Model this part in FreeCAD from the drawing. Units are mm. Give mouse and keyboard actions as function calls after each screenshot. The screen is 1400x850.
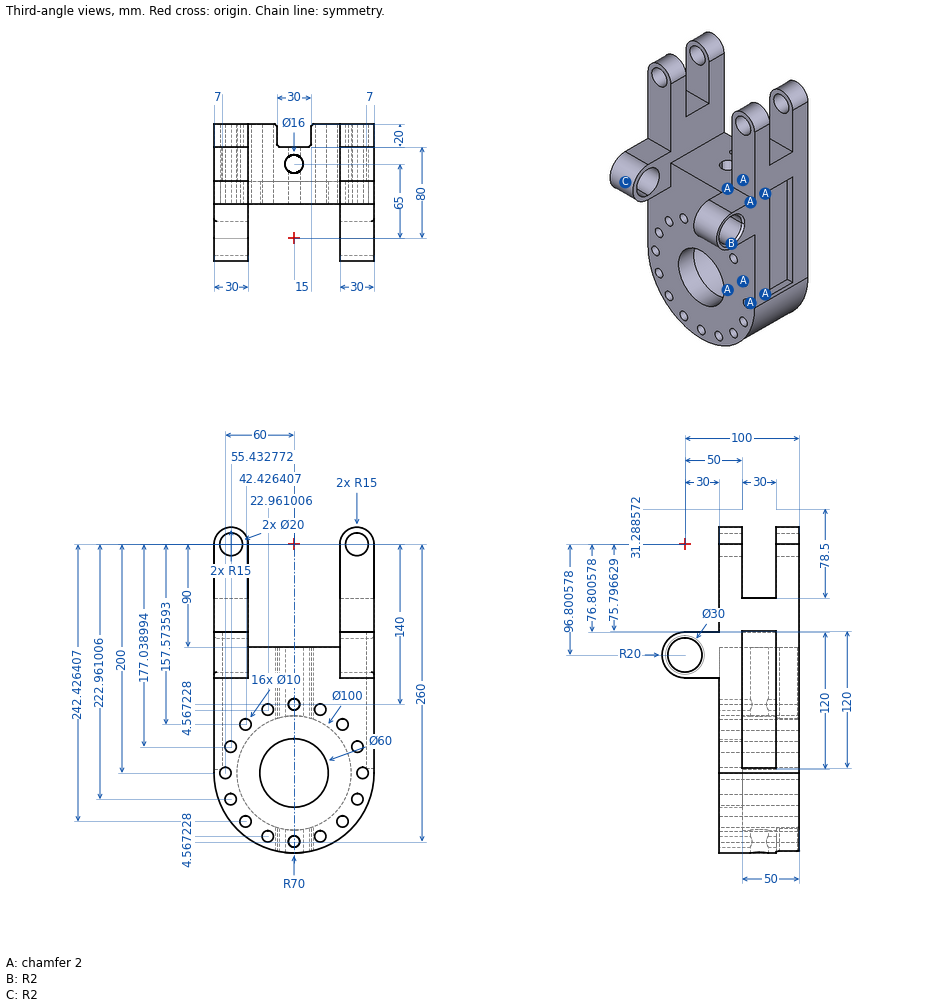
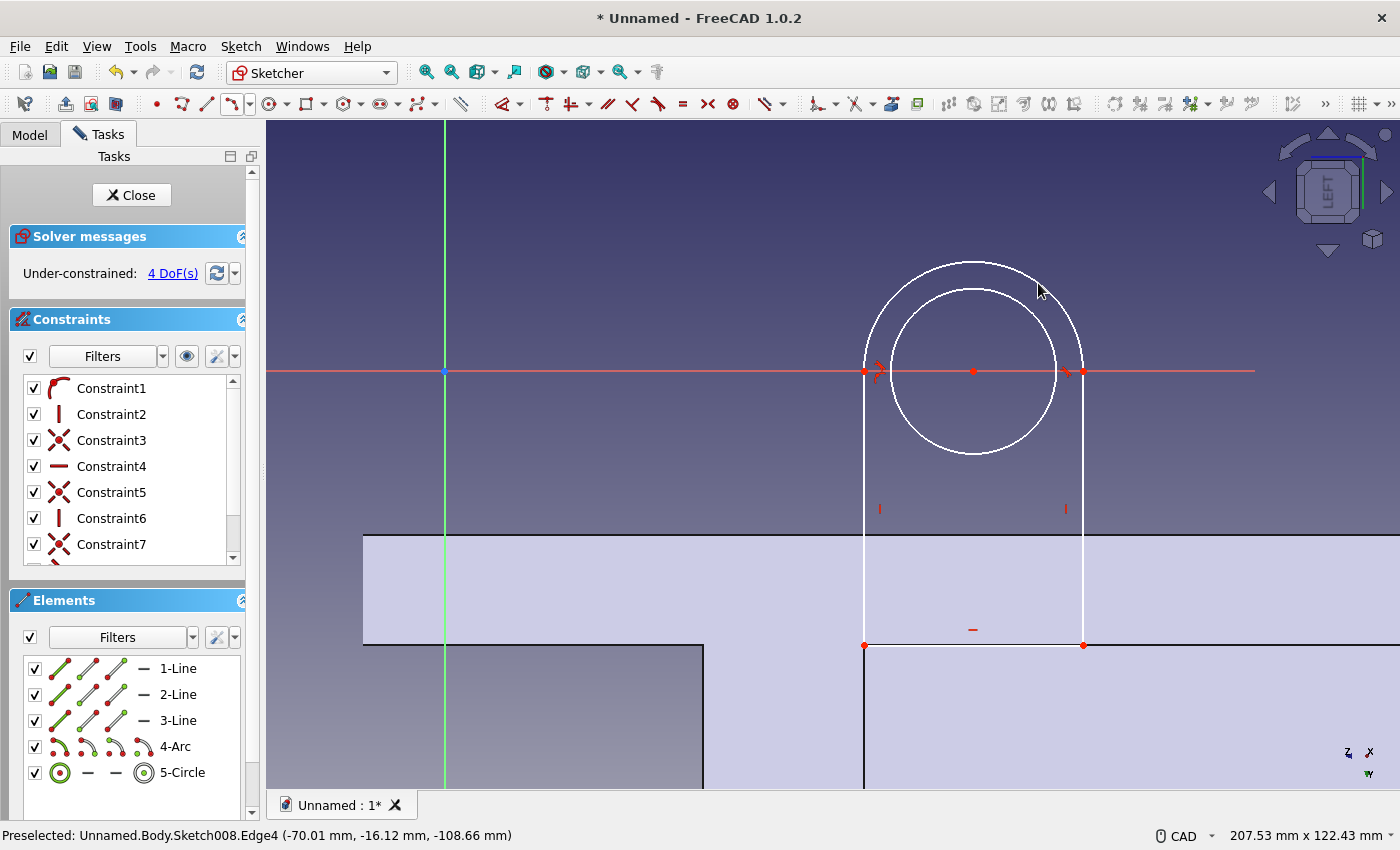
click(502, 104)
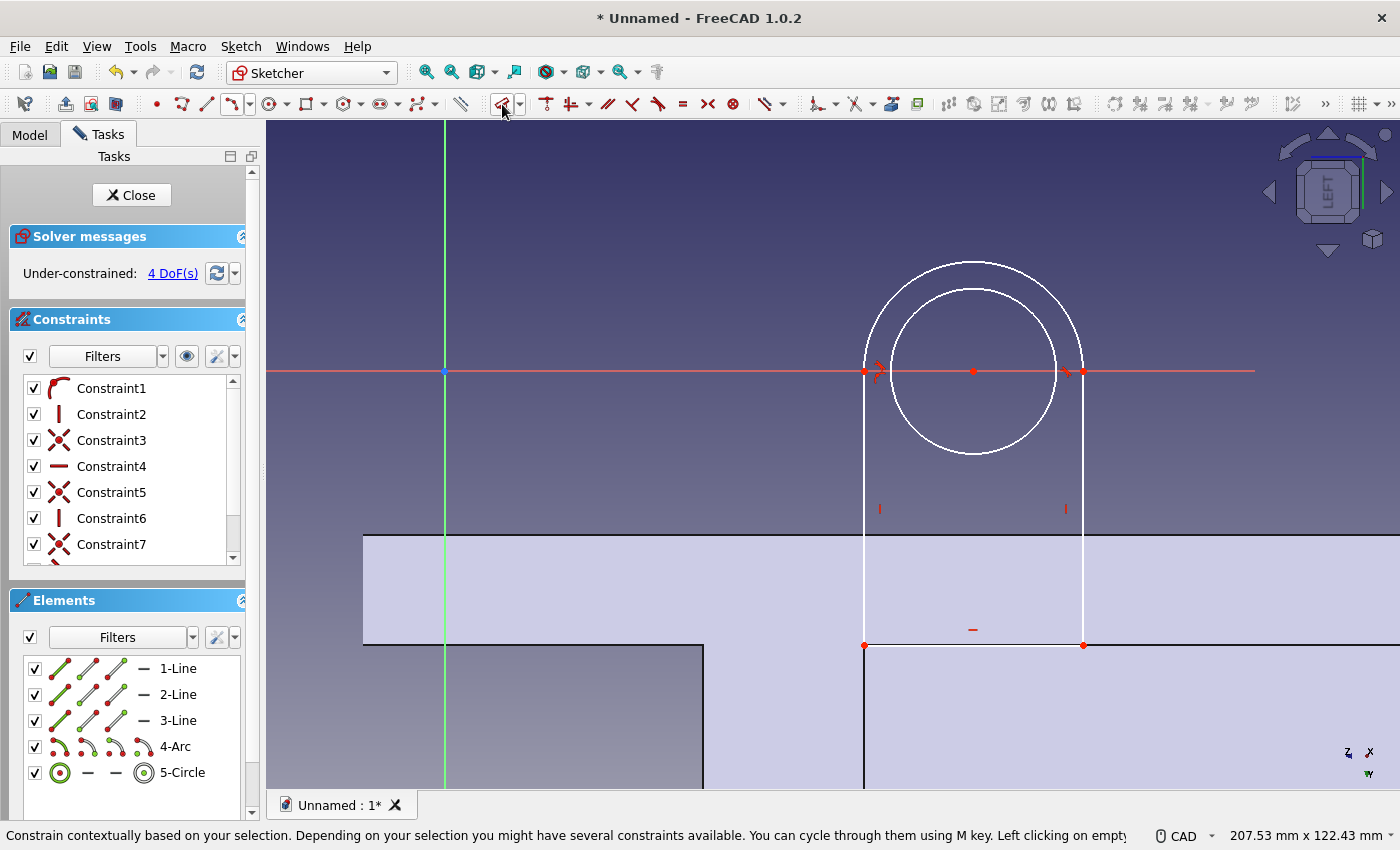
click(1038, 283)
click(1057, 257)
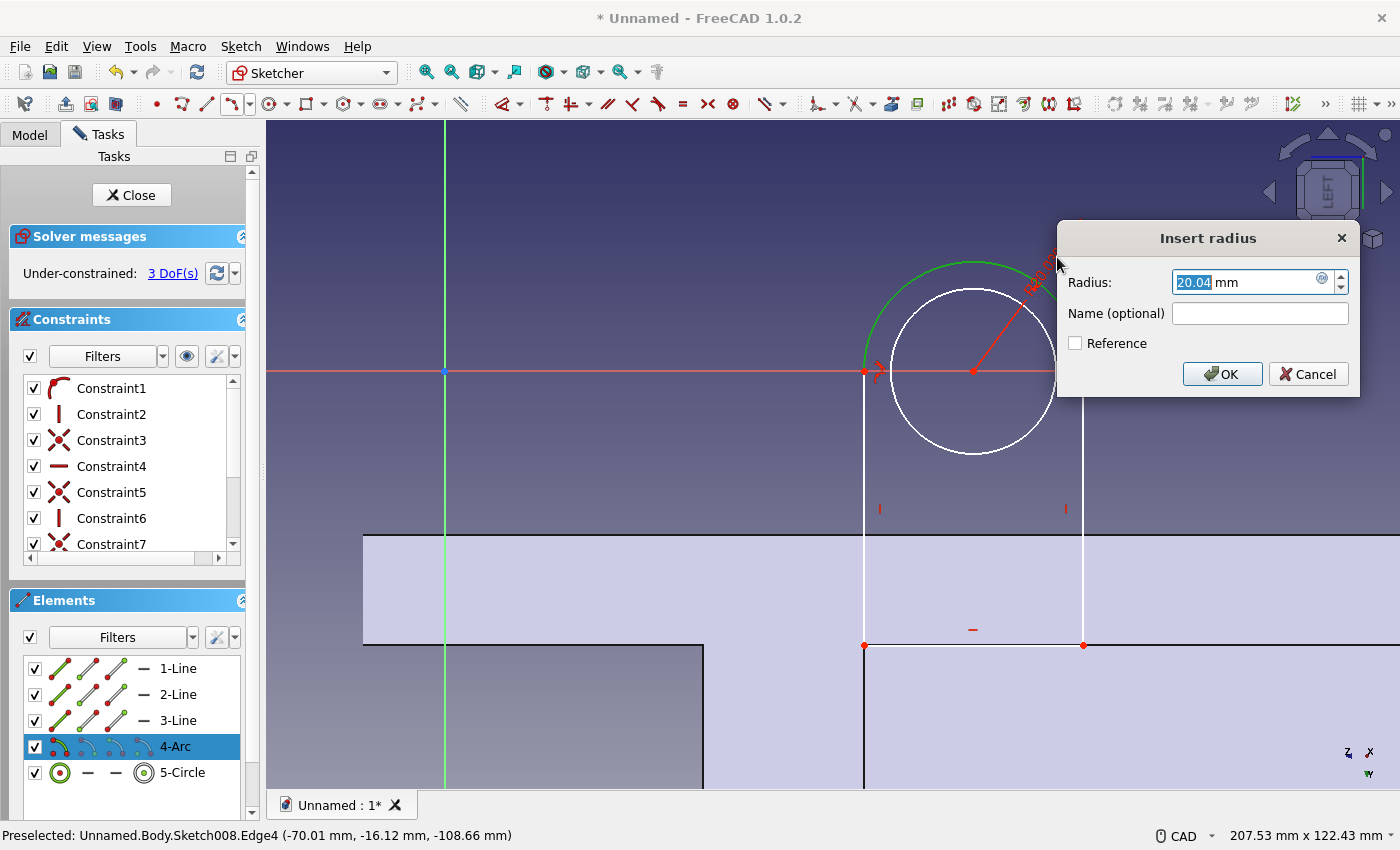
text(20)
key(Return)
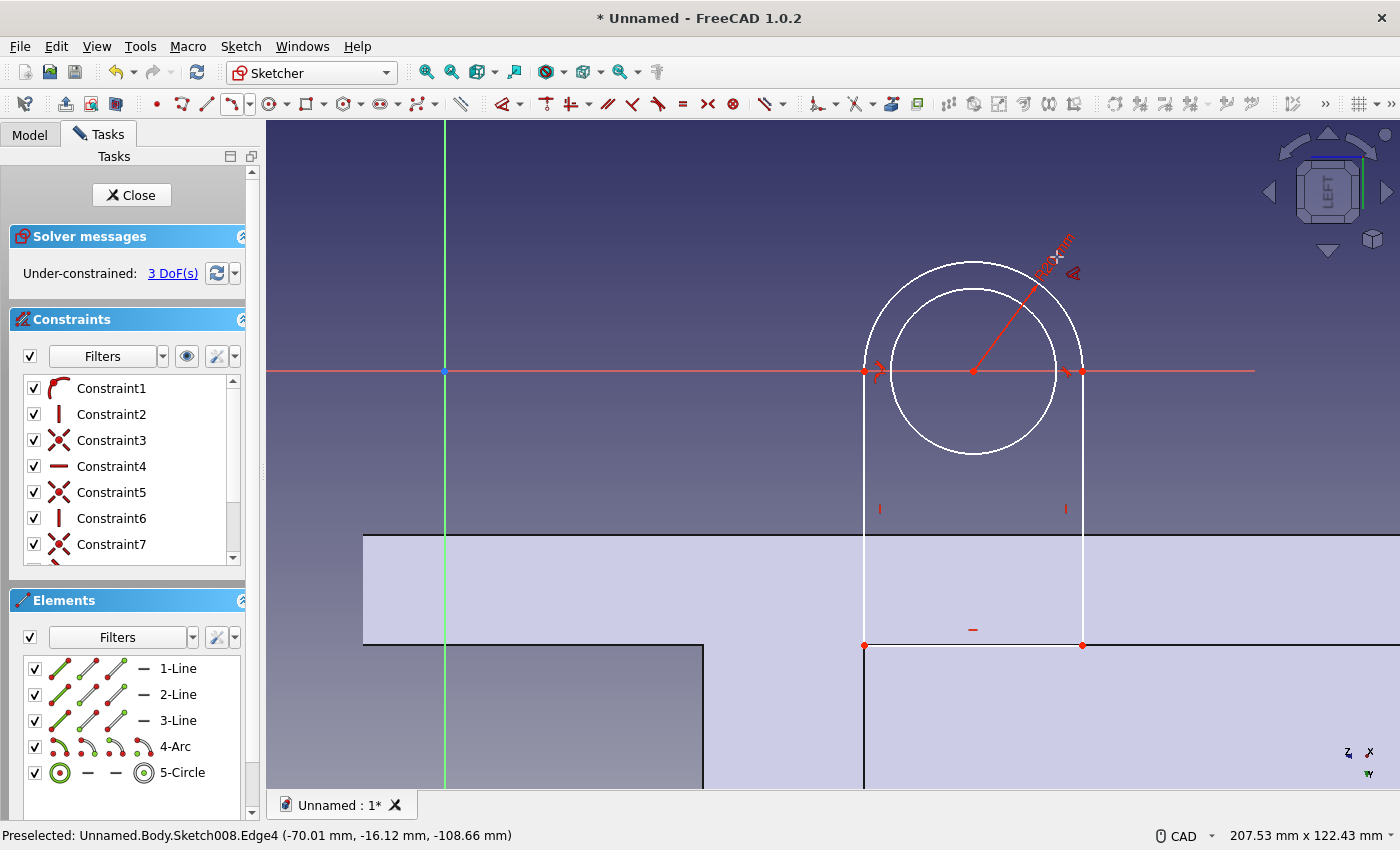
click(1032, 313)
click(1055, 452)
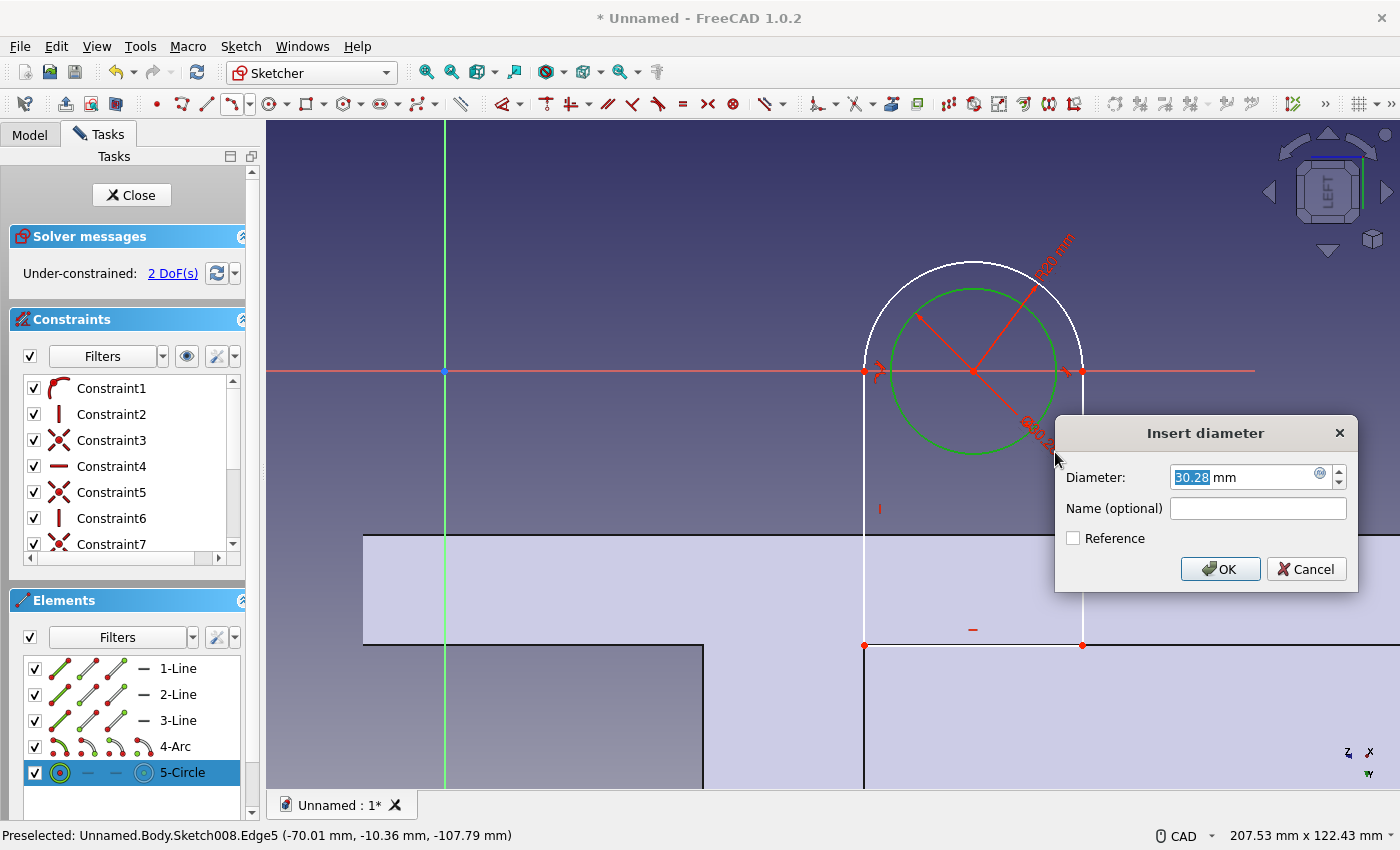
text(30)
key(Return)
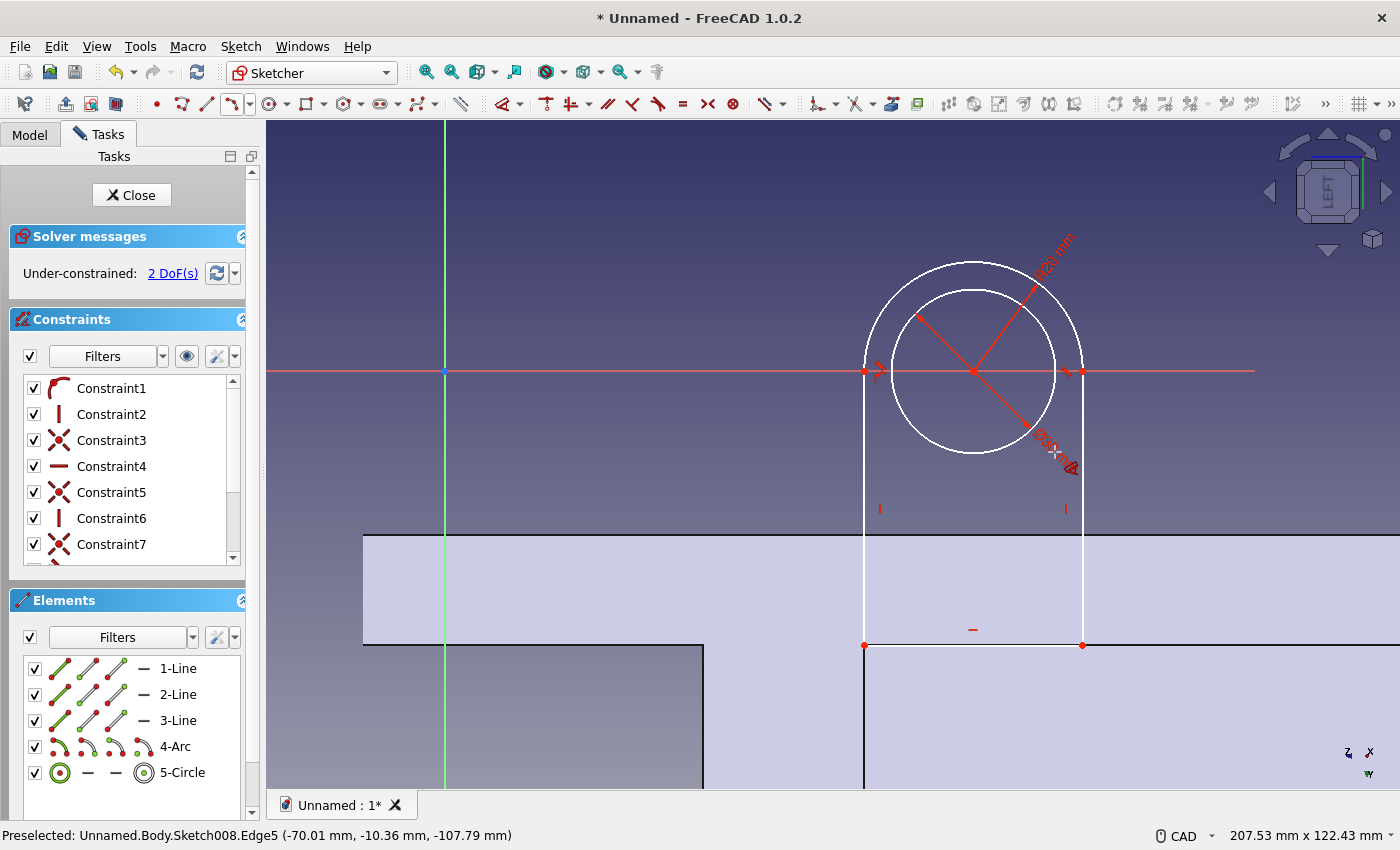
click(864, 454)
click(898, 509)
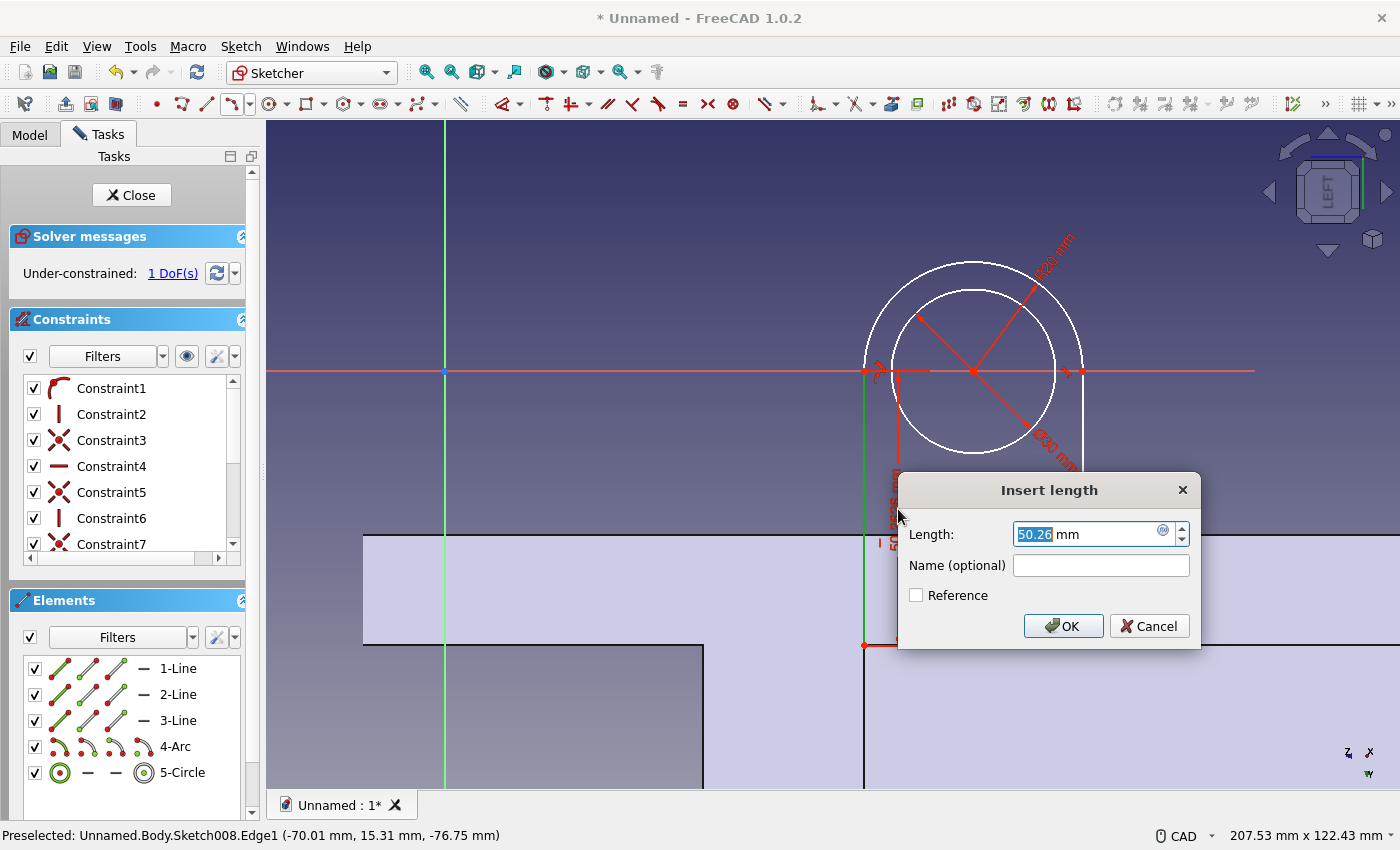
text(50)
key(Return)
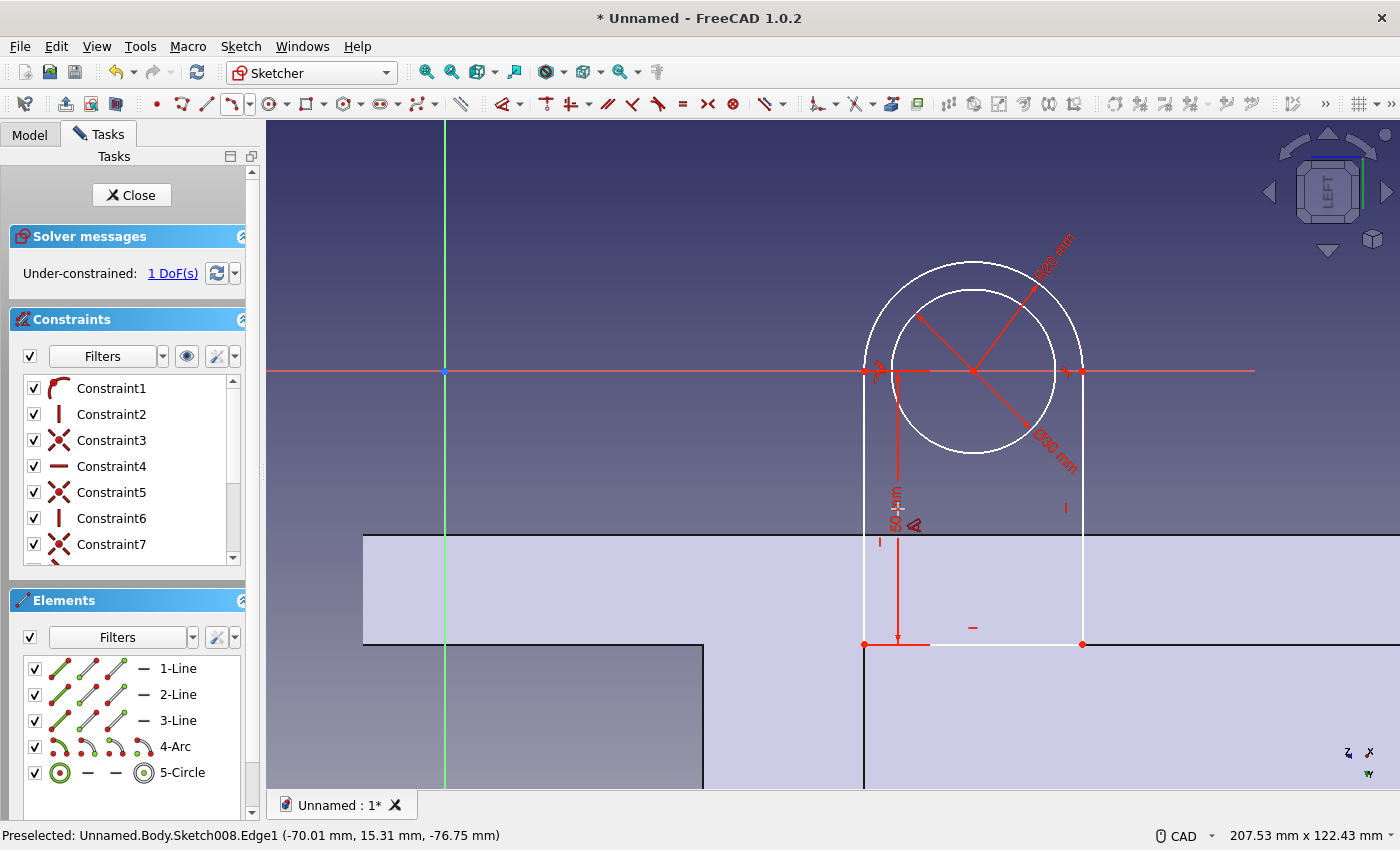
click(973, 371)
click(709, 337)